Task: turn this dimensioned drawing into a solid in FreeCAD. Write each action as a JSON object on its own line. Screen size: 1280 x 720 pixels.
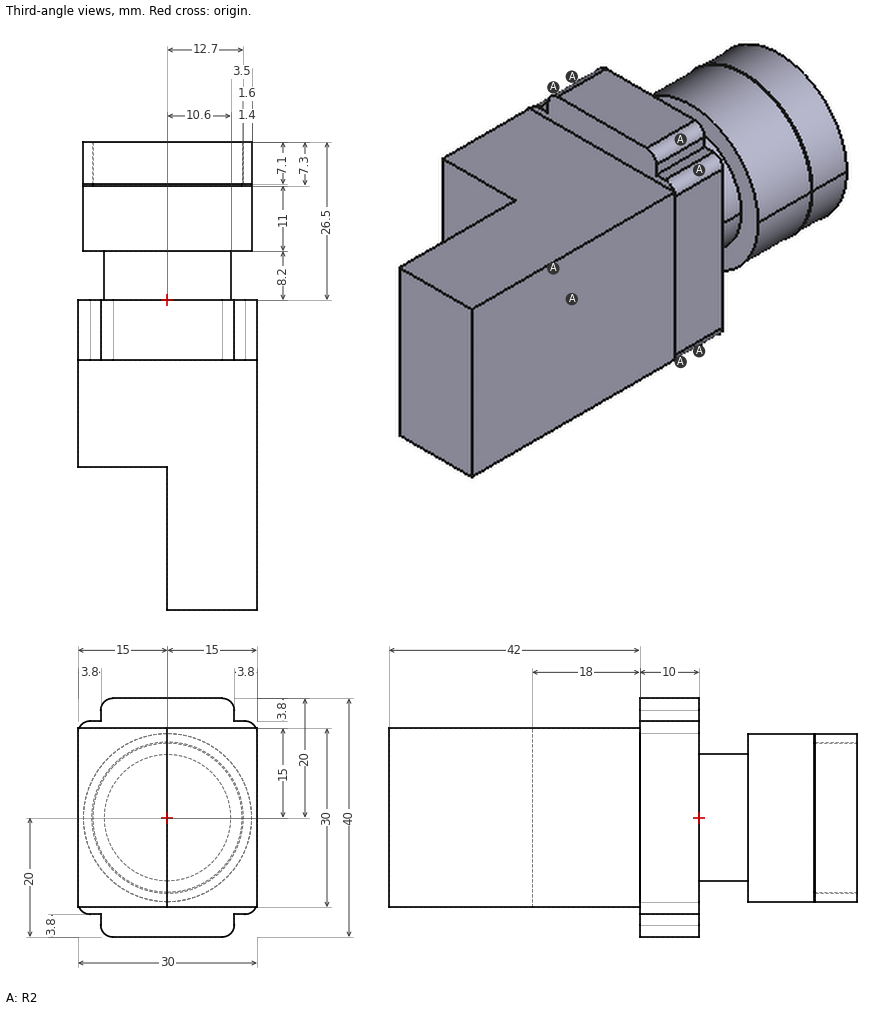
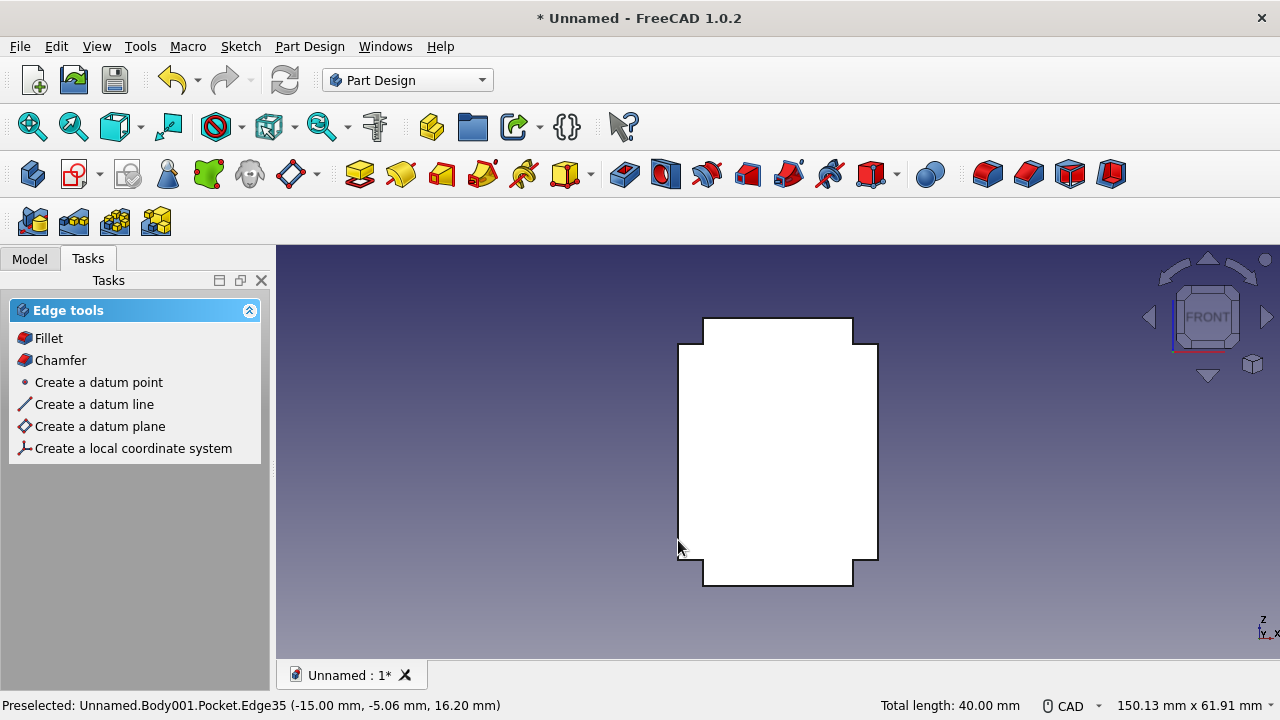
{"action": "key", "text": "3"}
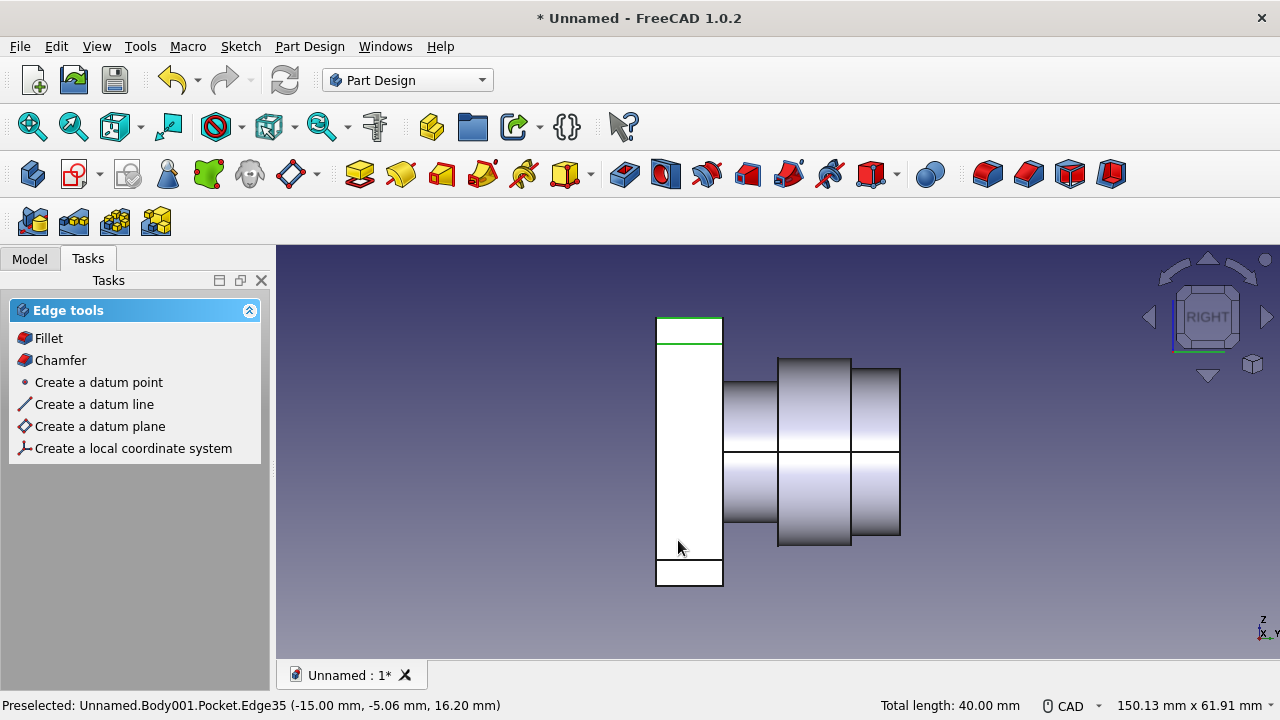
{"action": "left_click", "coordinate": [689, 585], "text": "ctrl"}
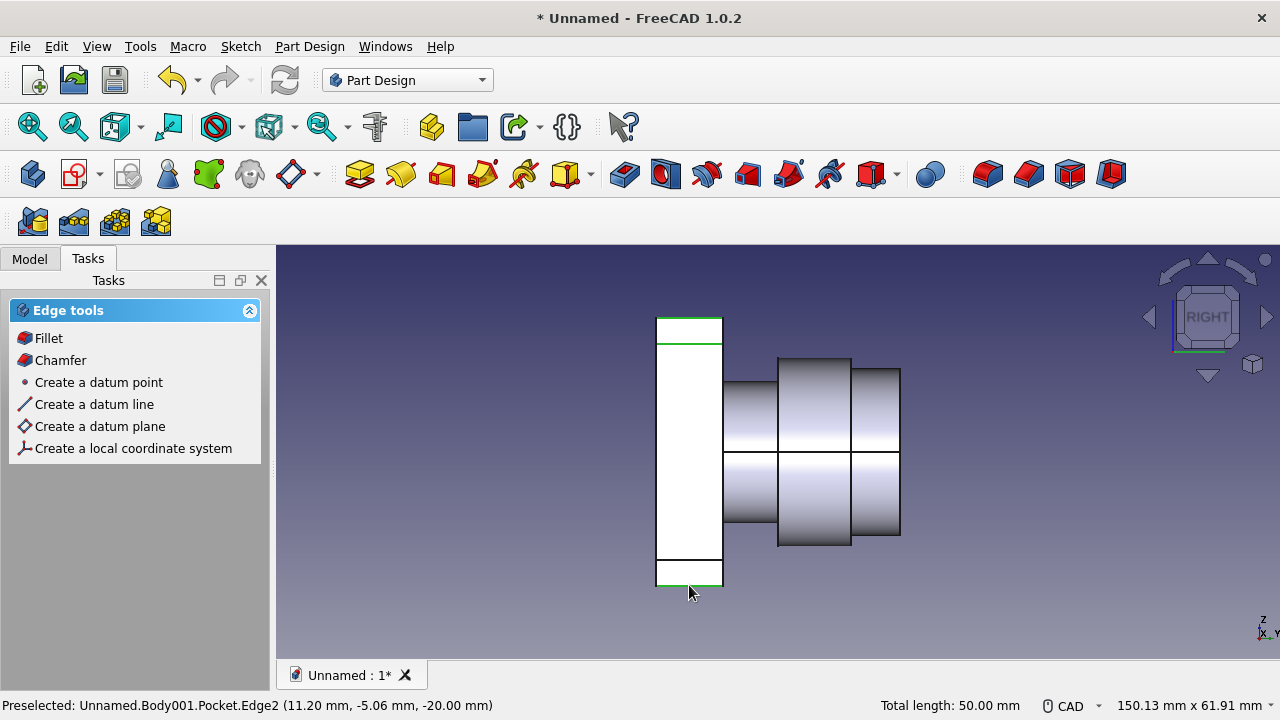
{"action": "left_click", "coordinate": [689, 559], "text": "ctrl"}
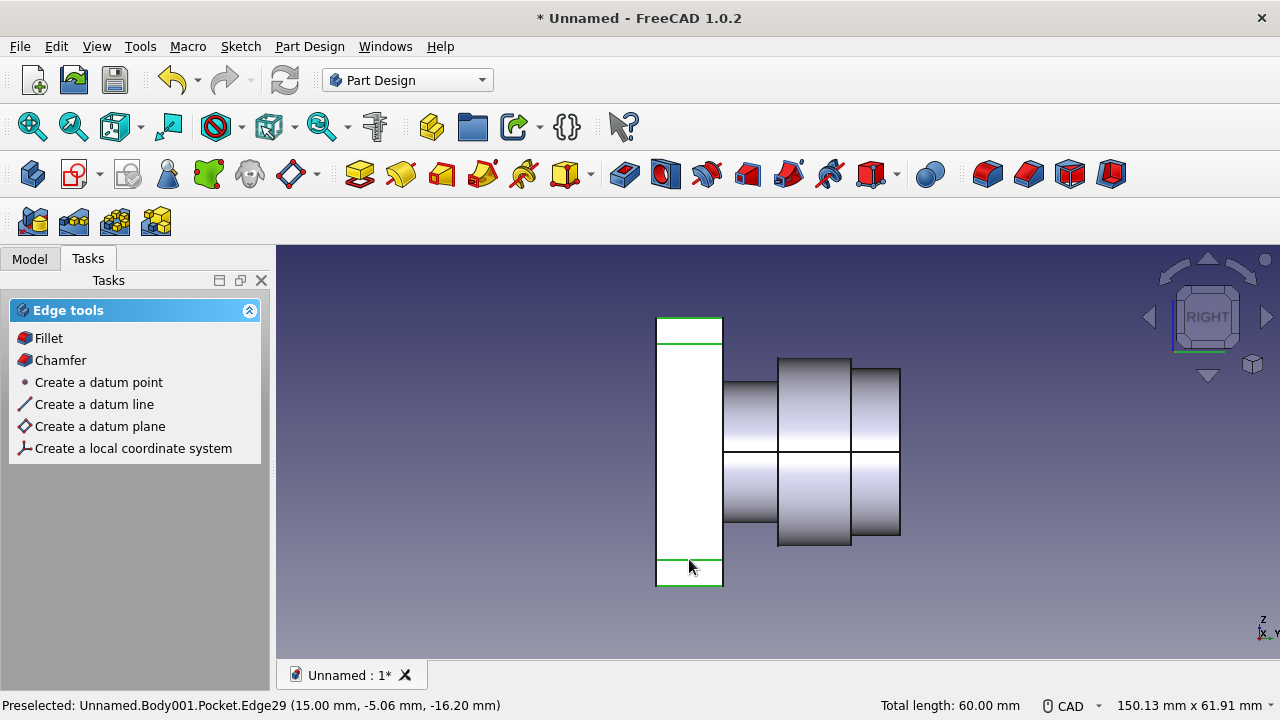
{"action": "key", "text": "5"}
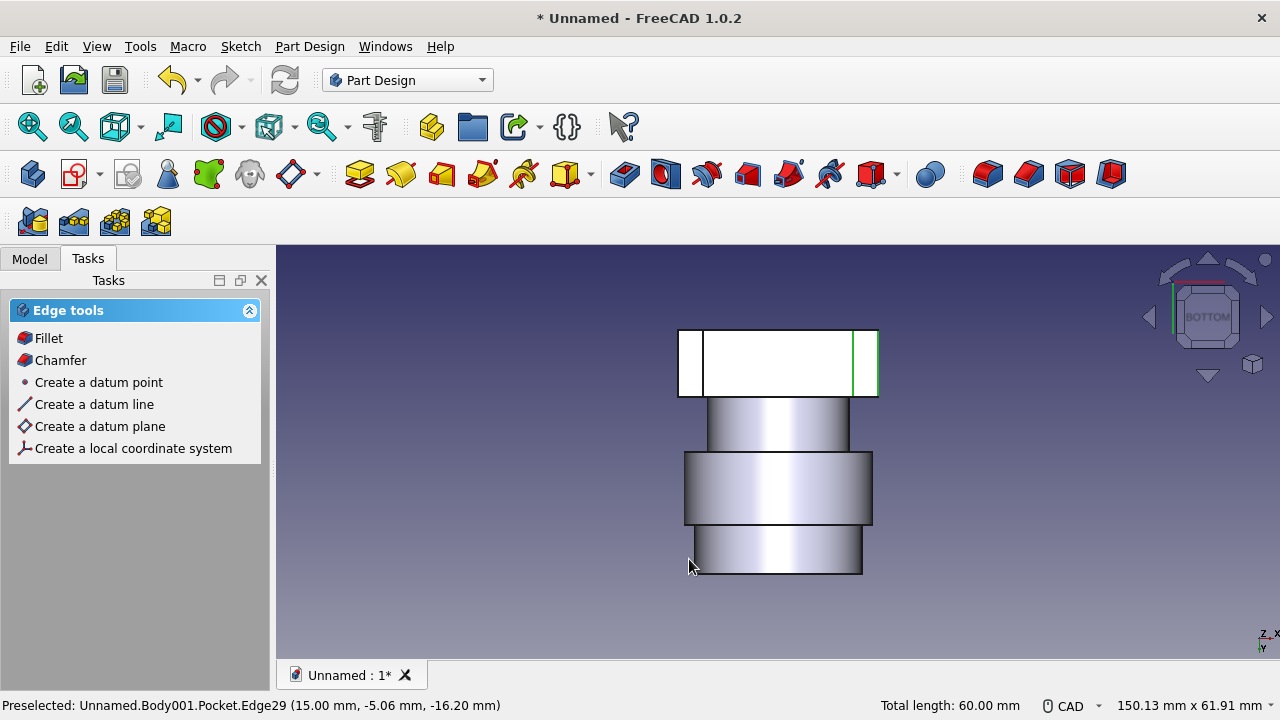
{"action": "key", "text": "v f"}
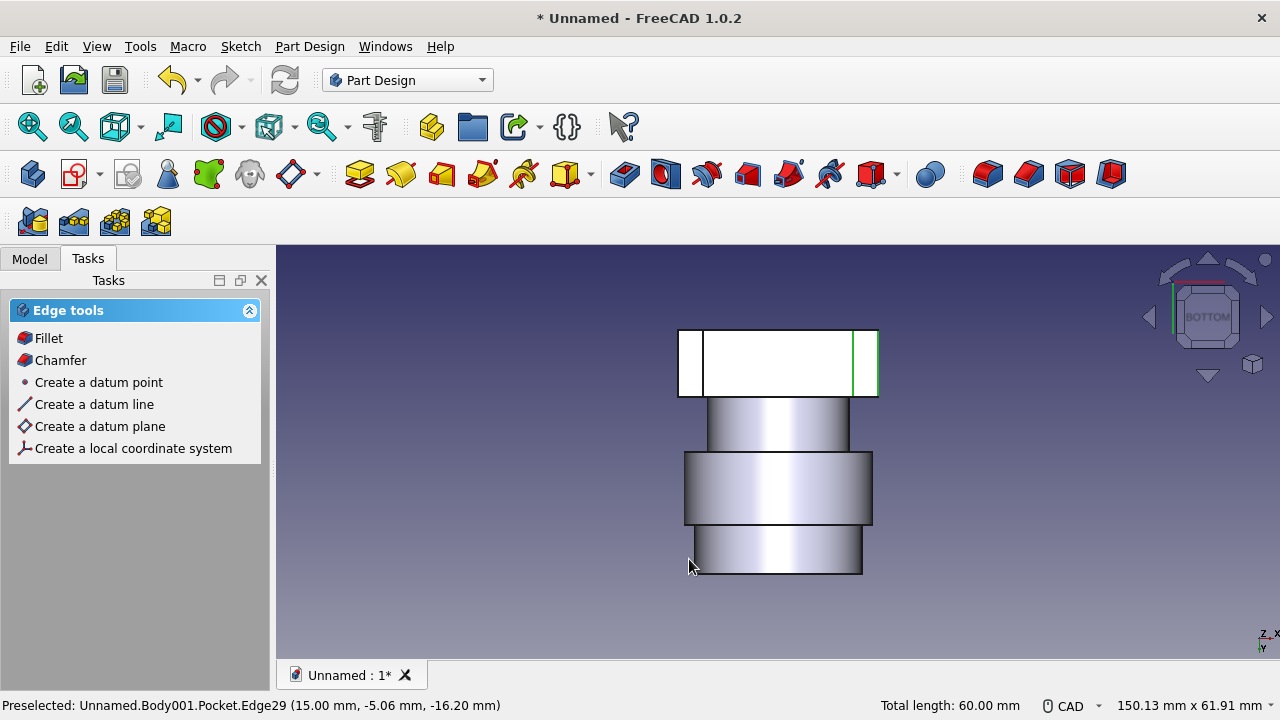
{"action": "left_click", "coordinate": [678, 362], "text": "ctrl"}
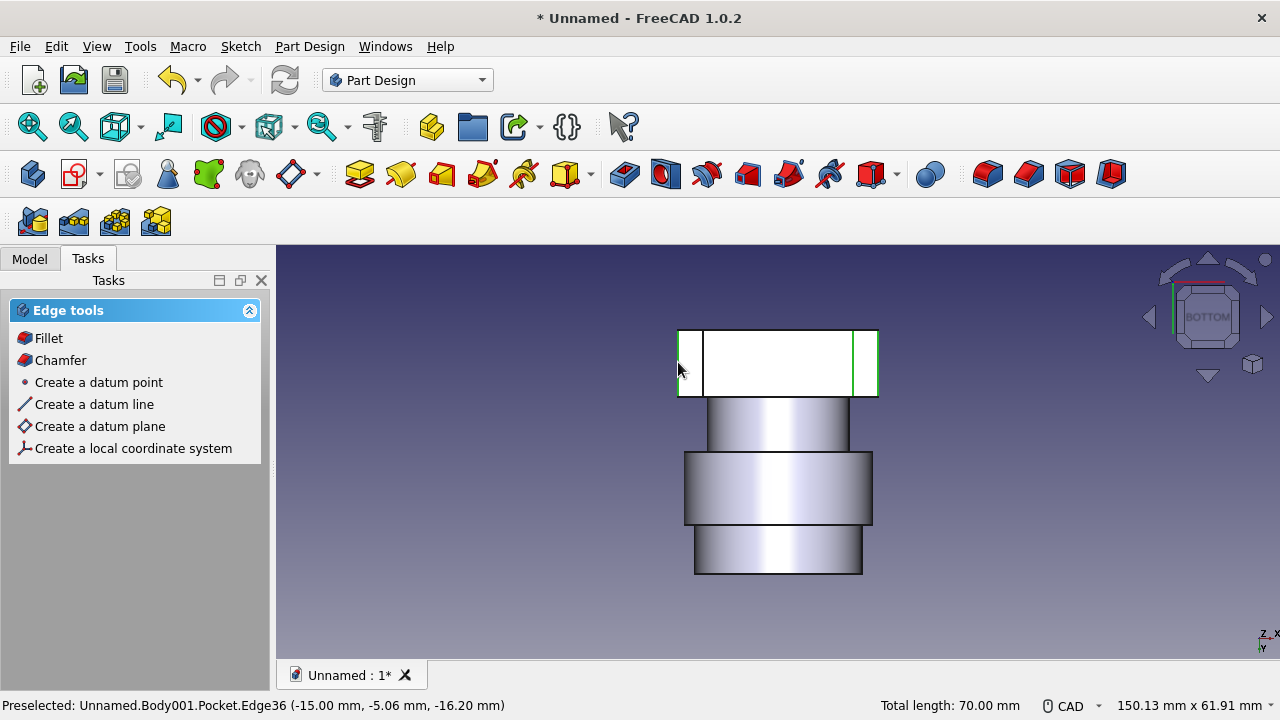
{"action": "left_click", "coordinate": [703, 362], "text": "ctrl"}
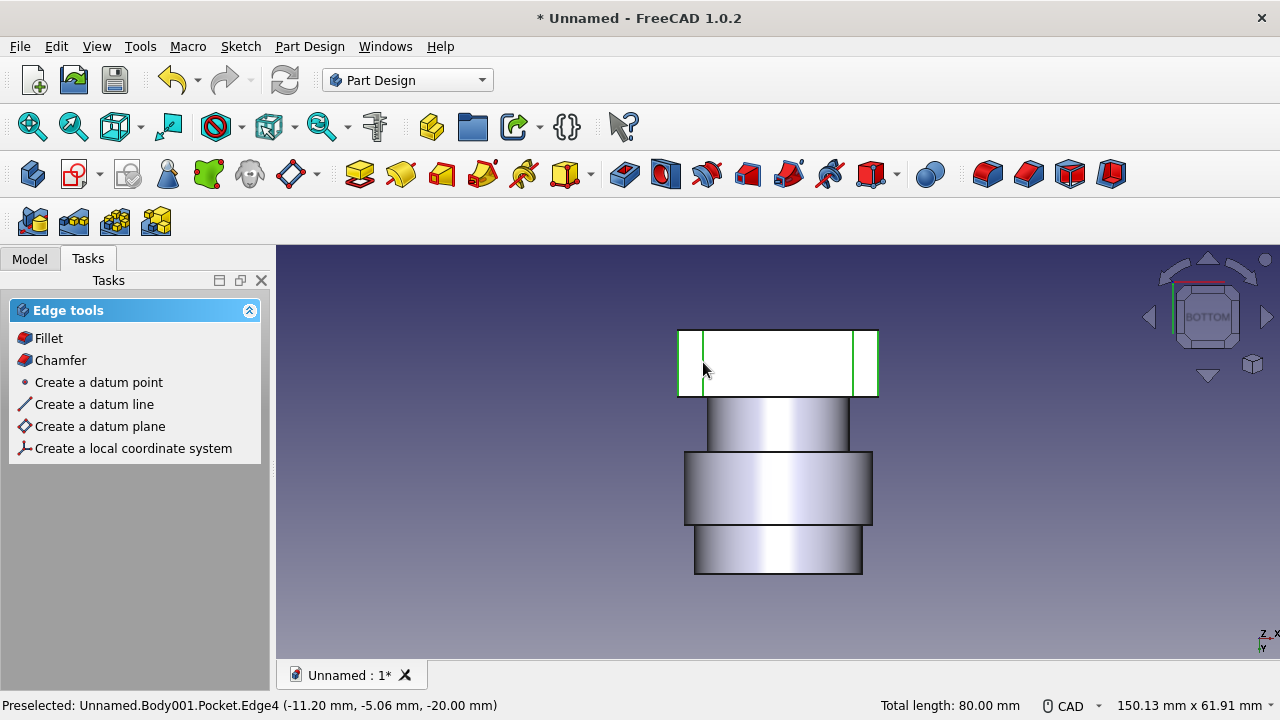
{"action": "left_click", "coordinate": [988, 174]}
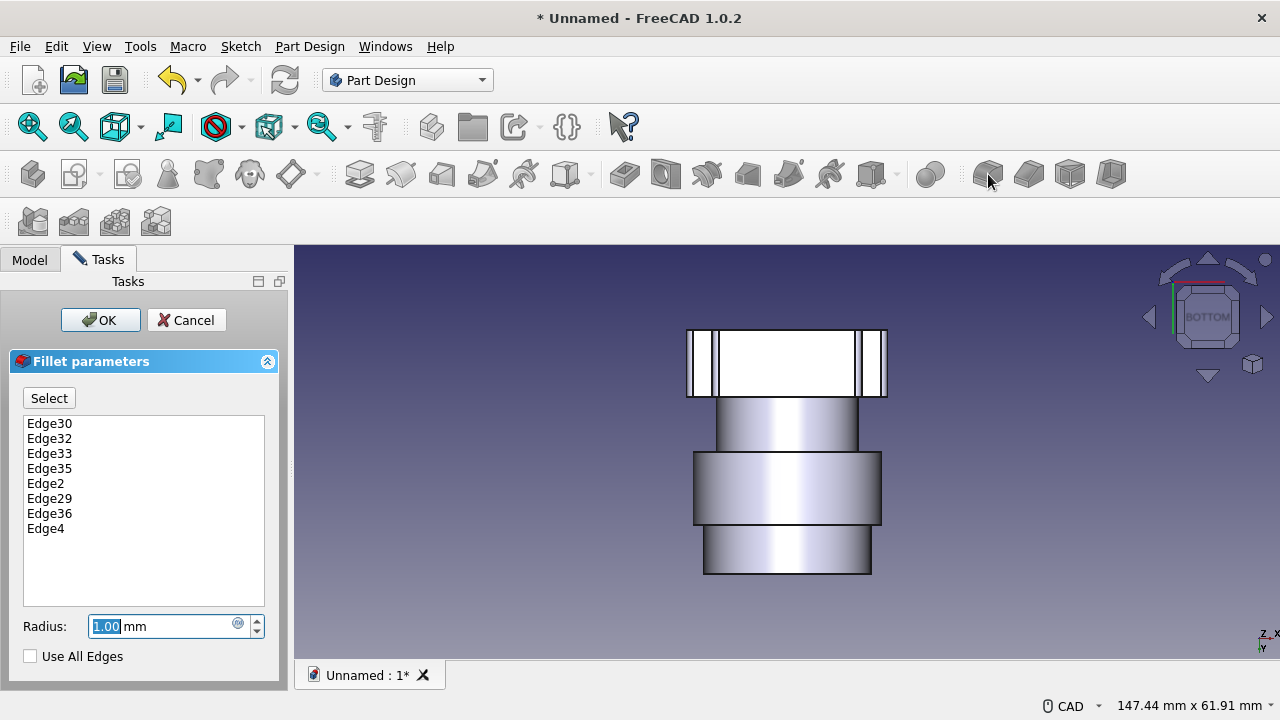
{"action": "type", "text": "2"}
{"action": "key", "text": "Tab"}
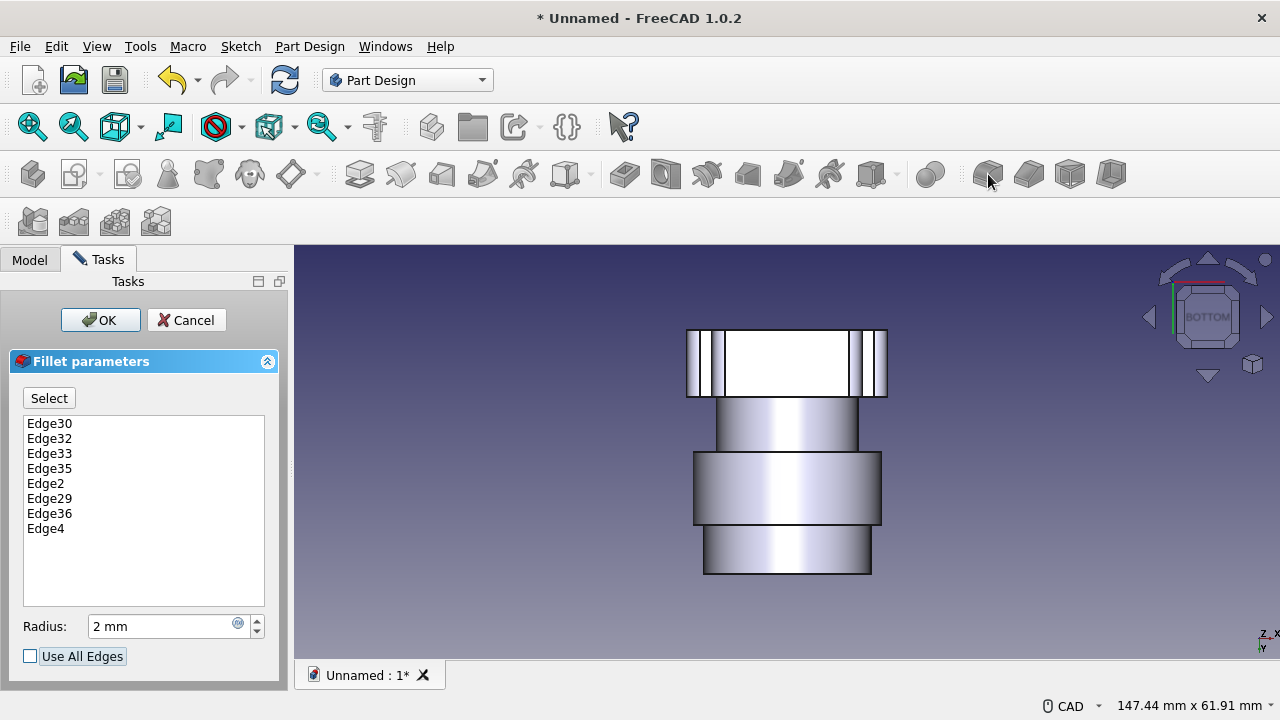
{"action": "left_click", "coordinate": [101, 320]}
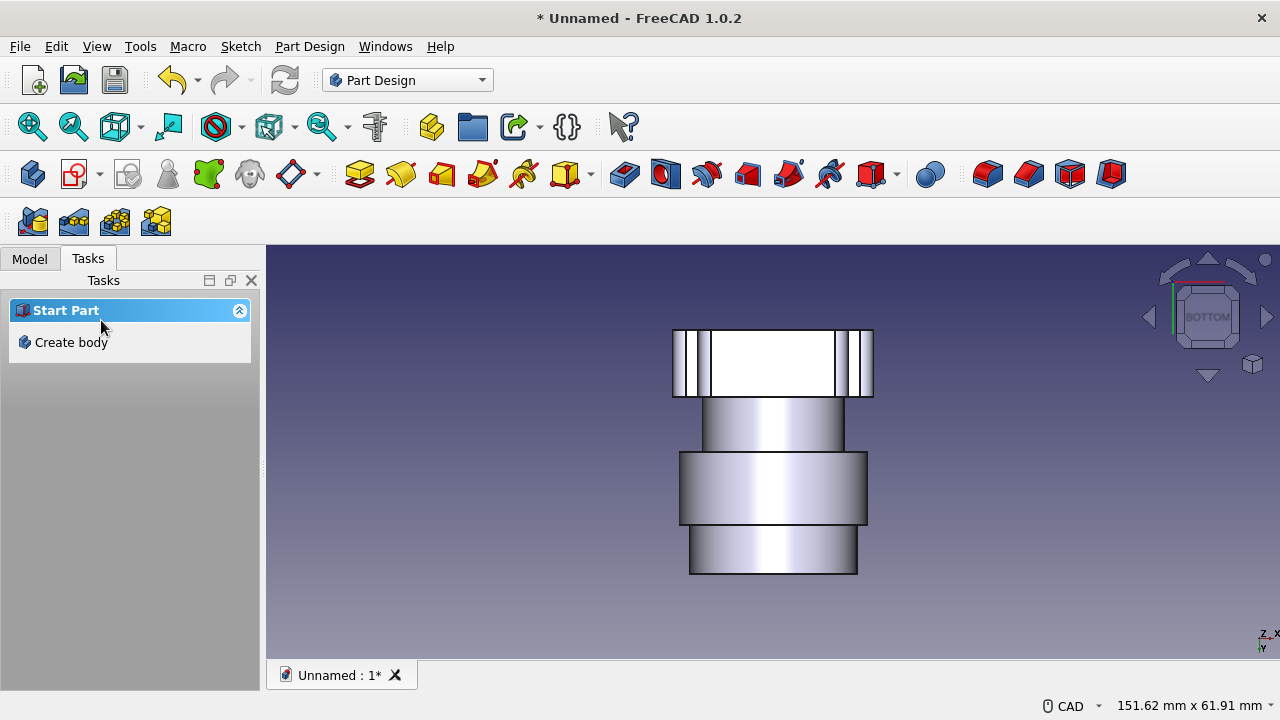
{"action": "key", "text": "v f"}